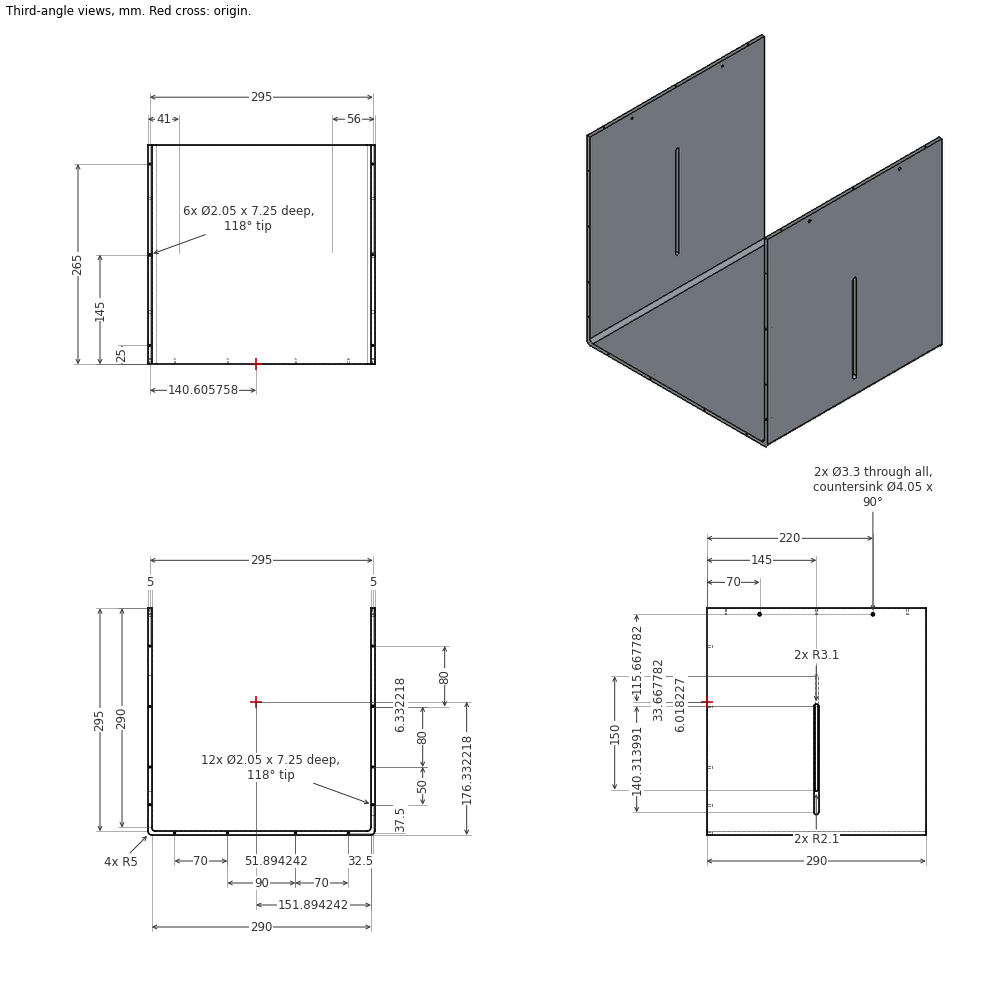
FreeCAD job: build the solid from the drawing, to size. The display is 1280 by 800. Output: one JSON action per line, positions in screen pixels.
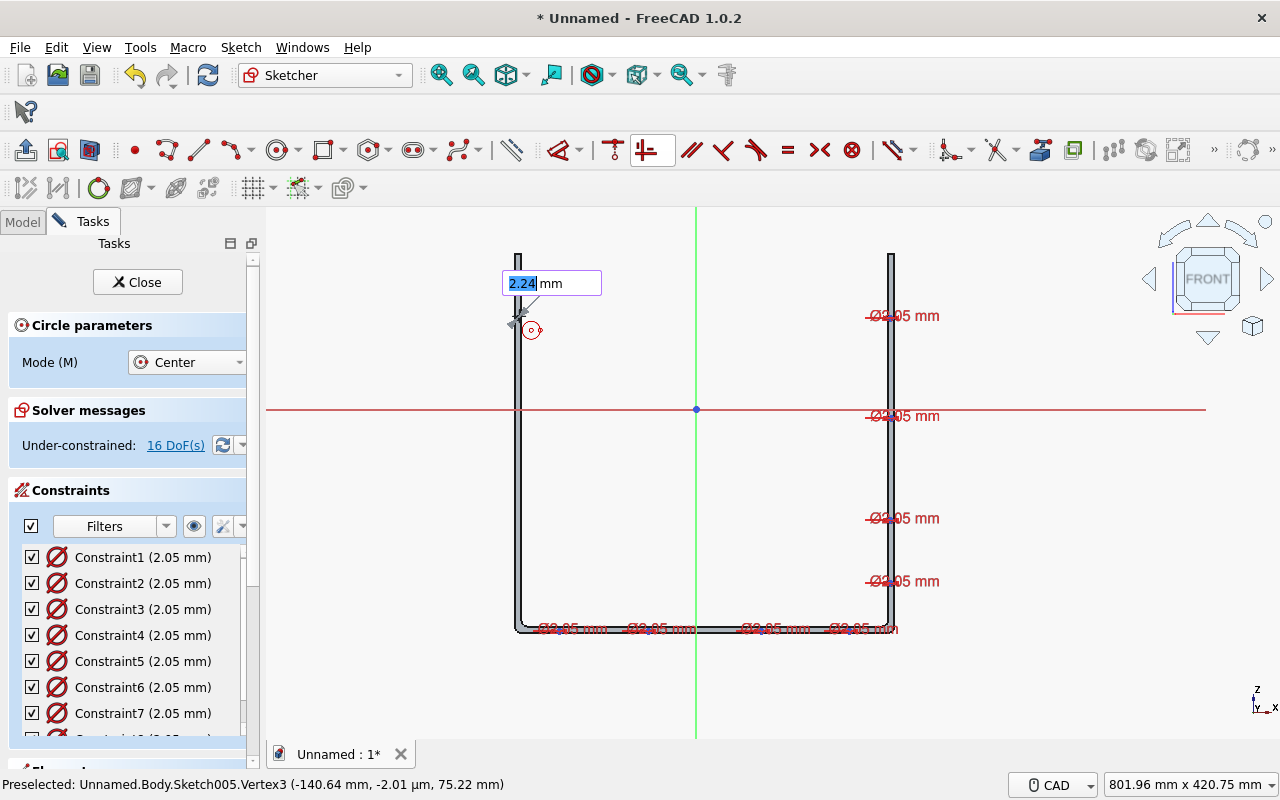
{"action": "type", "text": "2.05"}
{"action": "key", "text": "Return"}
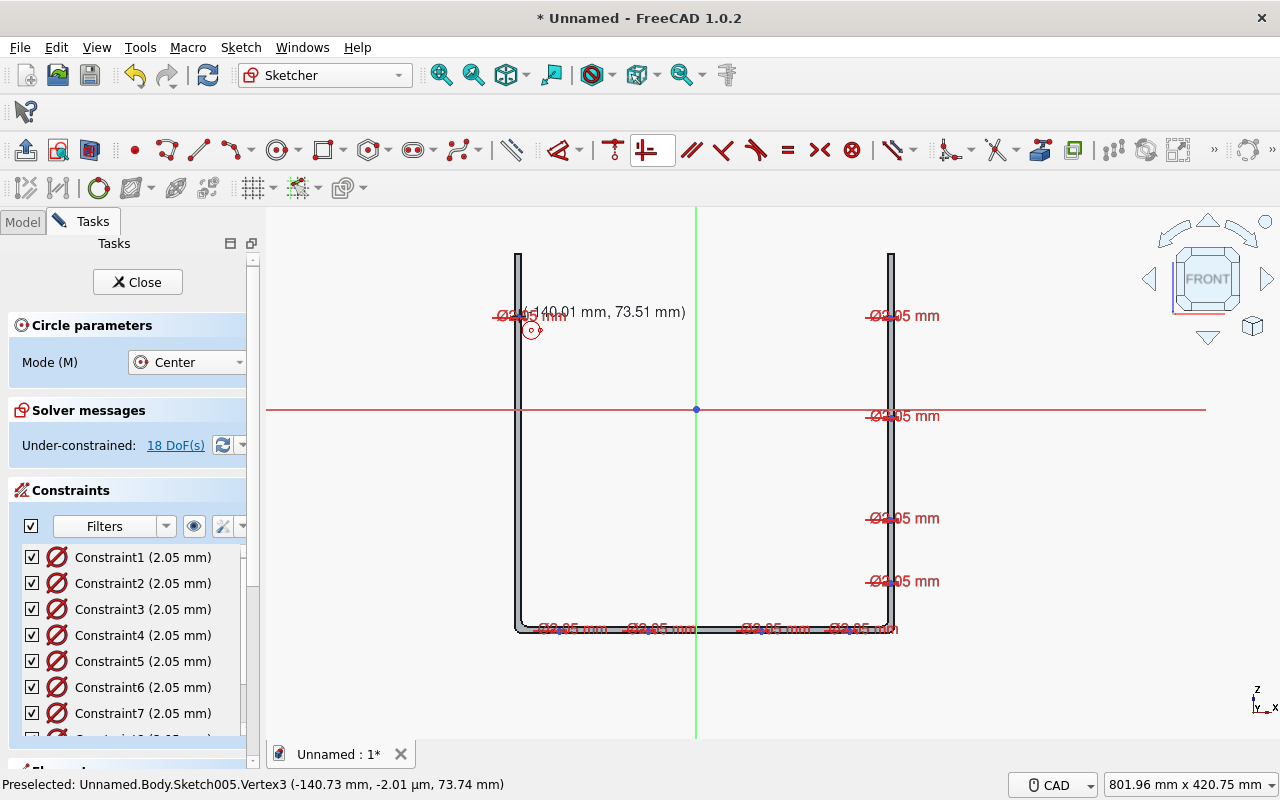
{"action": "scroll", "coordinate": [518, 418], "scroll_direction": "up", "scroll_amount": 15}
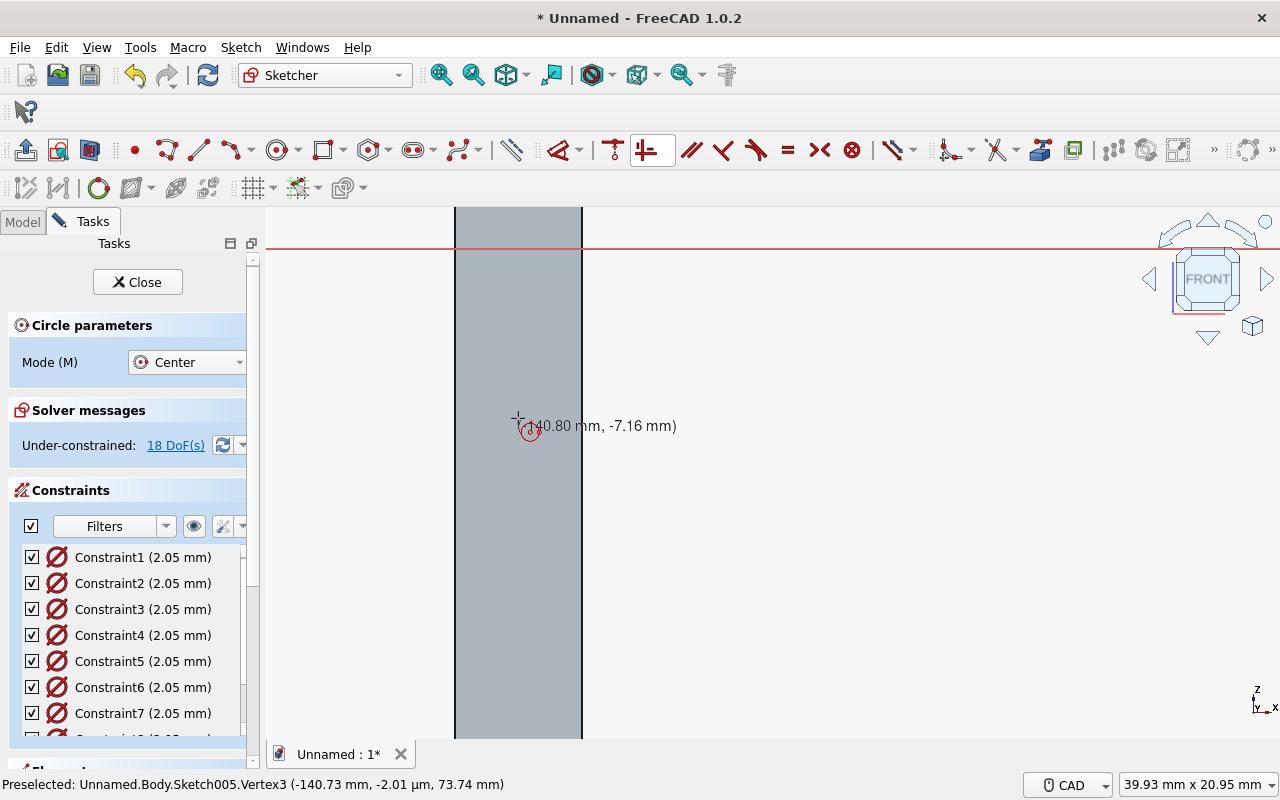
{"action": "scroll", "coordinate": [518, 418], "scroll_direction": "down", "scroll_amount": 15}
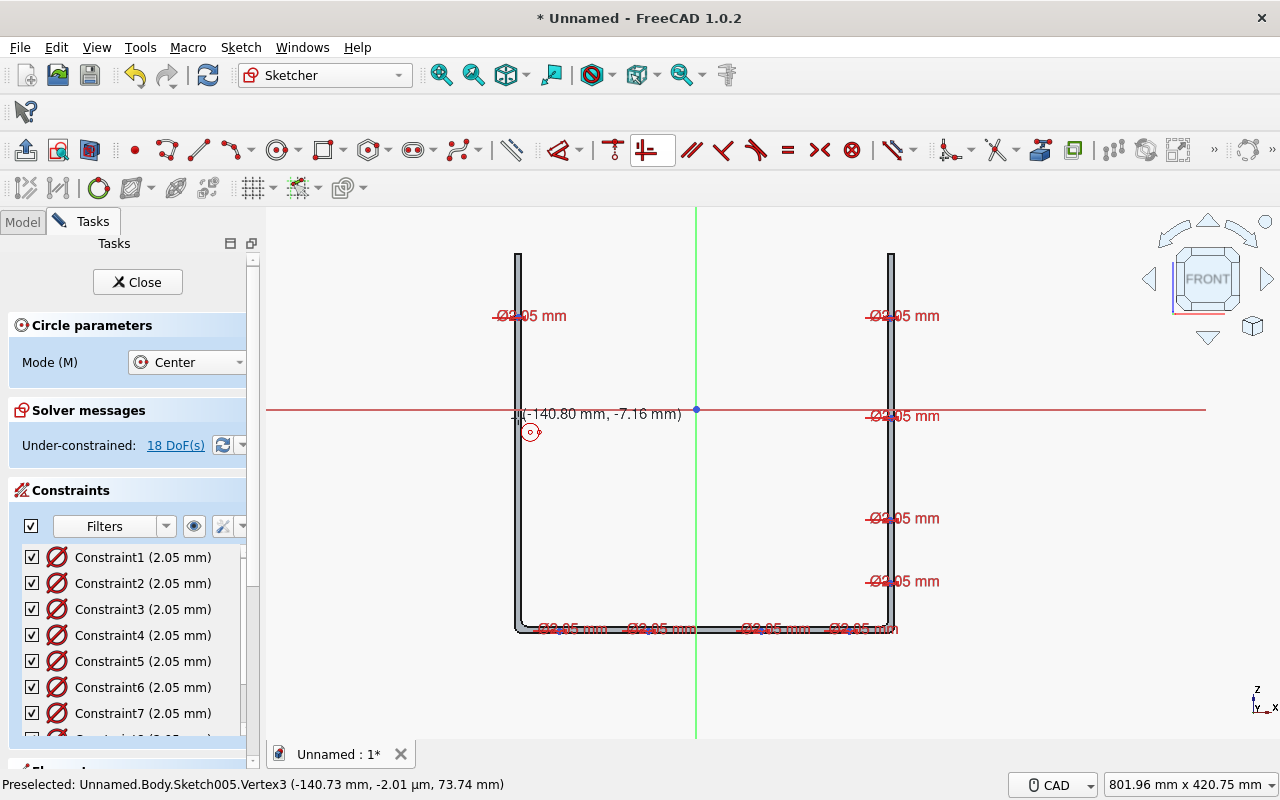
{"action": "scroll", "coordinate": [518, 418], "scroll_direction": "up", "scroll_amount": 4}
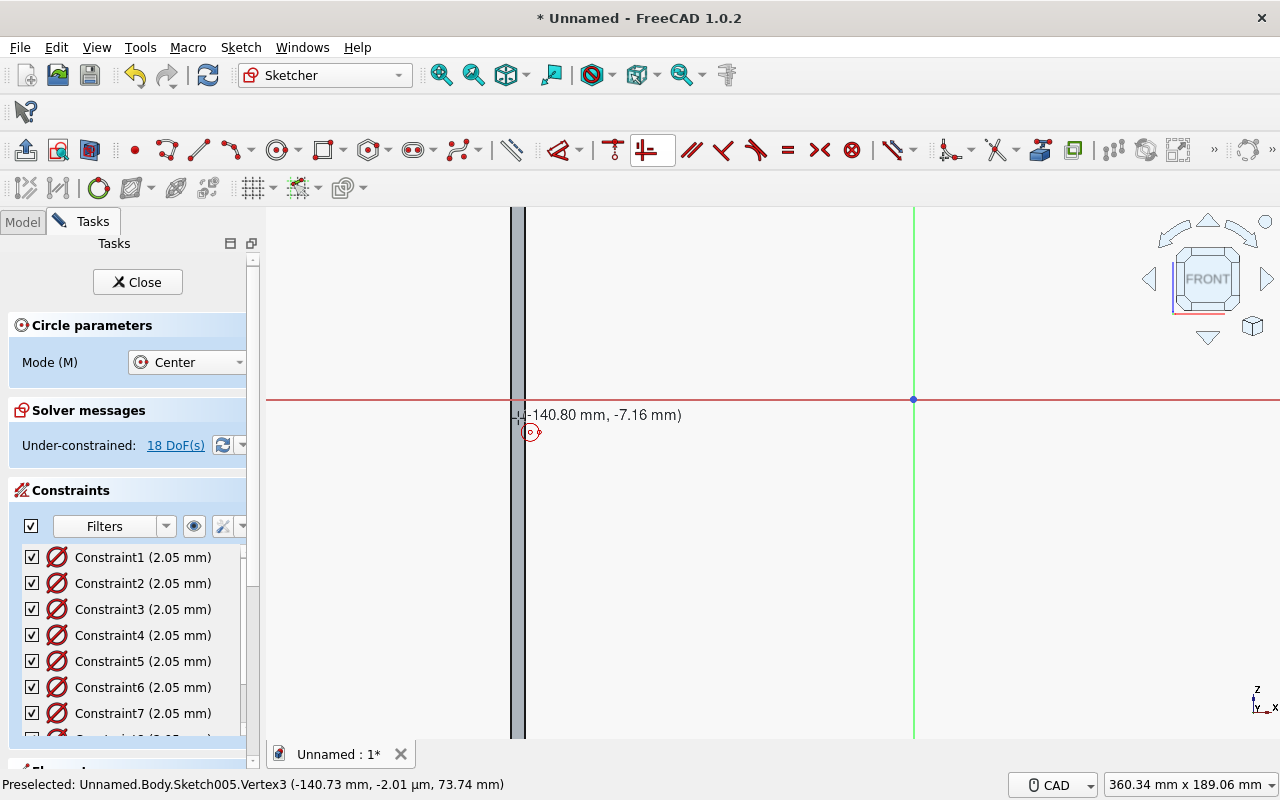
{"action": "left_click", "coordinate": [518, 417]}
{"action": "mouse_move", "coordinate": [520, 415]}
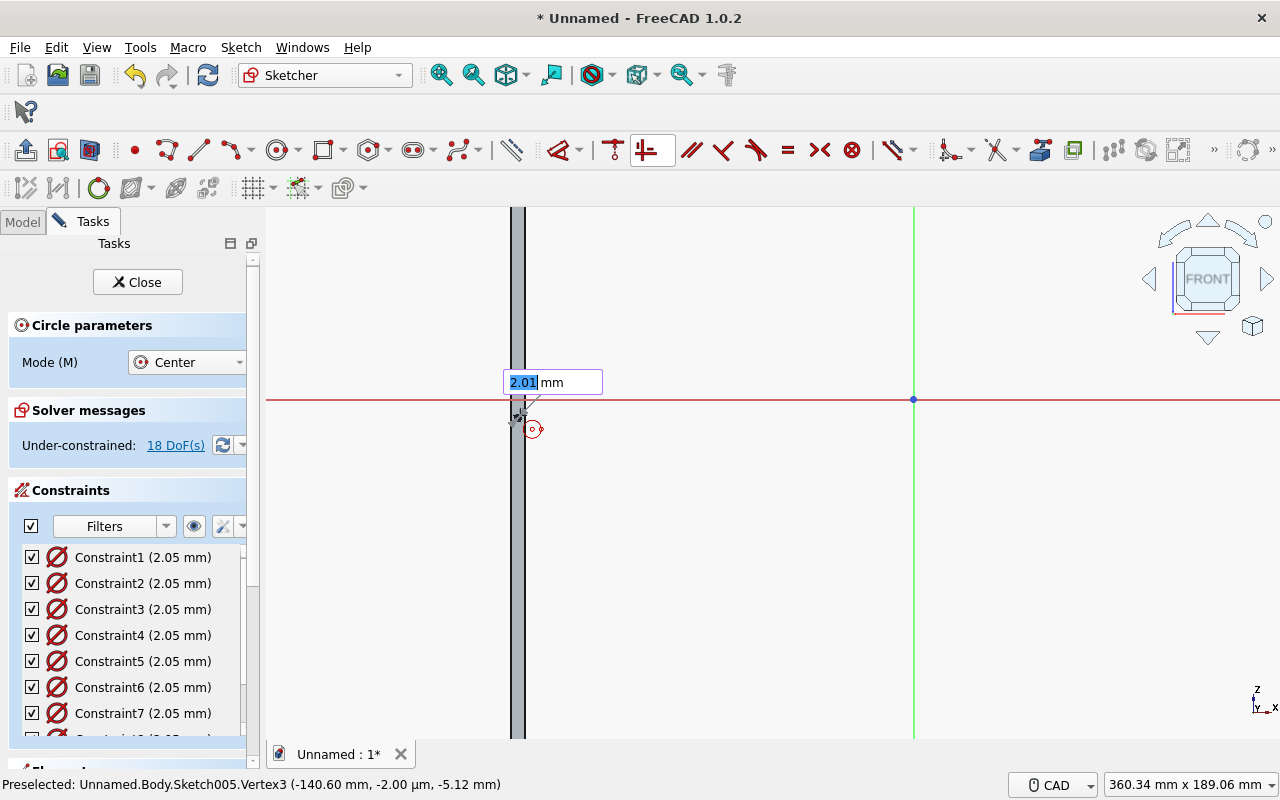
{"action": "type", "text": "2.05"}
{"action": "key", "text": "Return"}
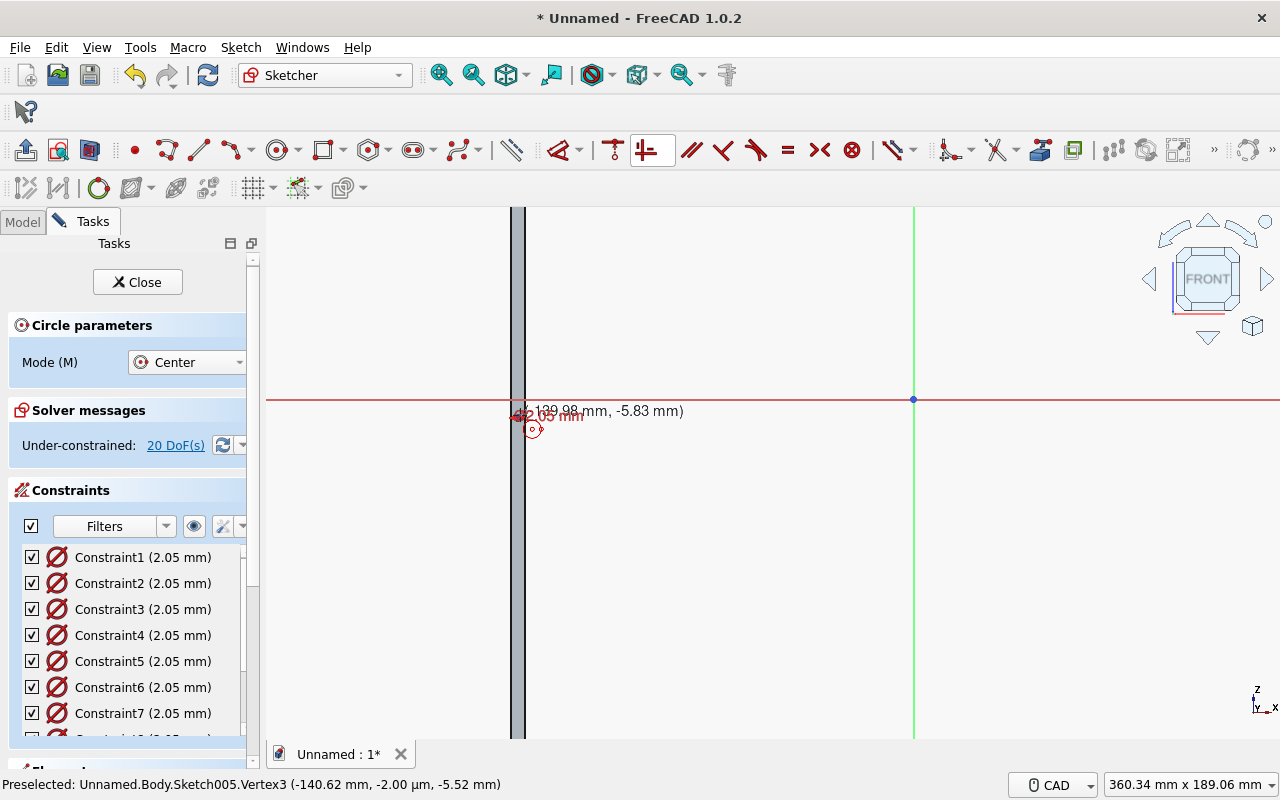
{"action": "scroll", "coordinate": [518, 643], "scroll_direction": "up", "scroll_amount": 11}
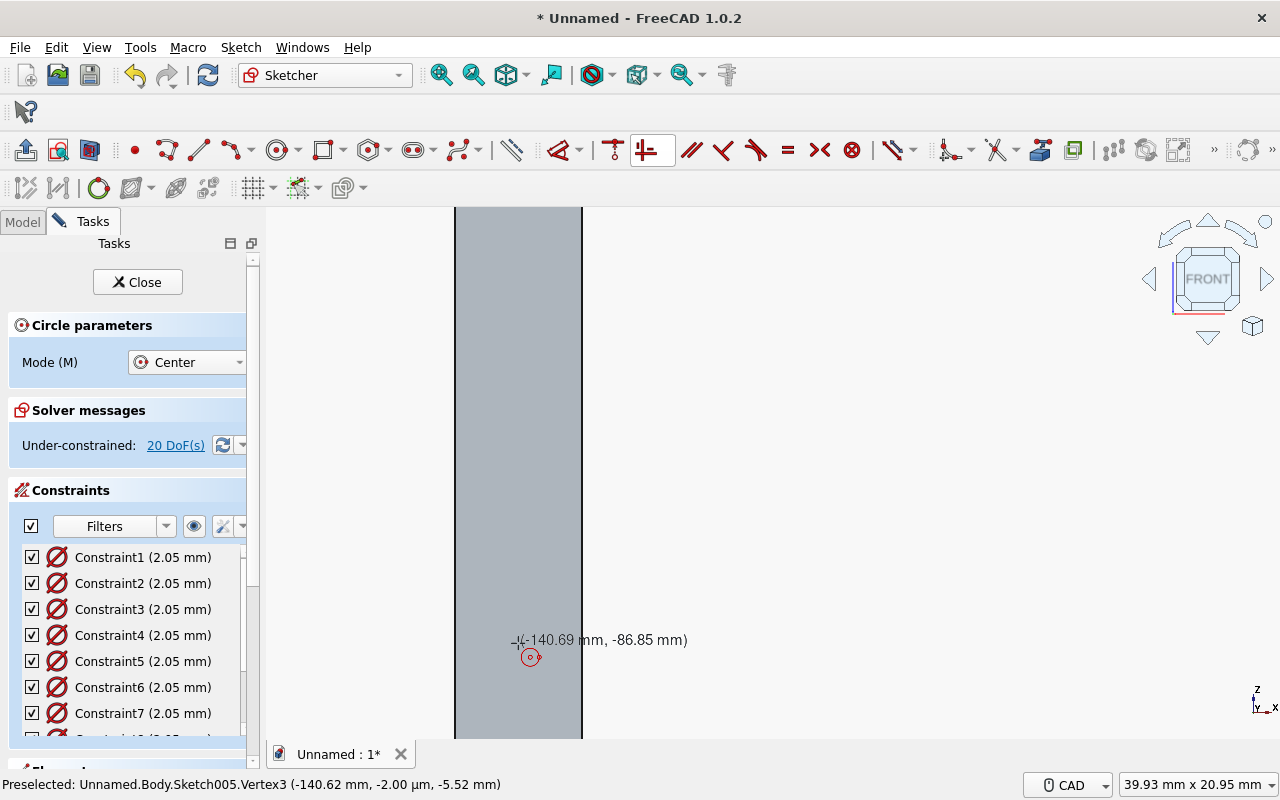
{"action": "scroll", "coordinate": [518, 513], "scroll_direction": "down", "scroll_amount": 15}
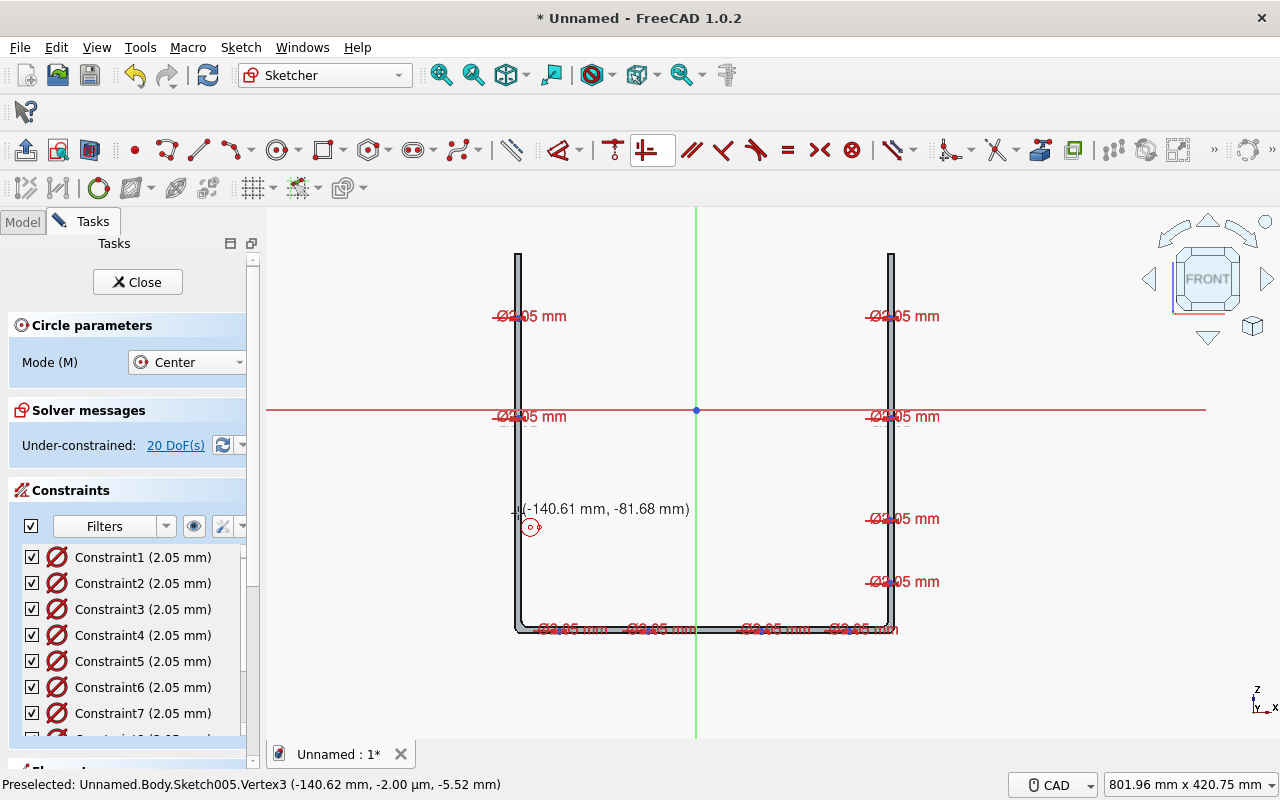
{"action": "left_click", "coordinate": [518, 519]}
{"action": "mouse_move", "coordinate": [519, 519]}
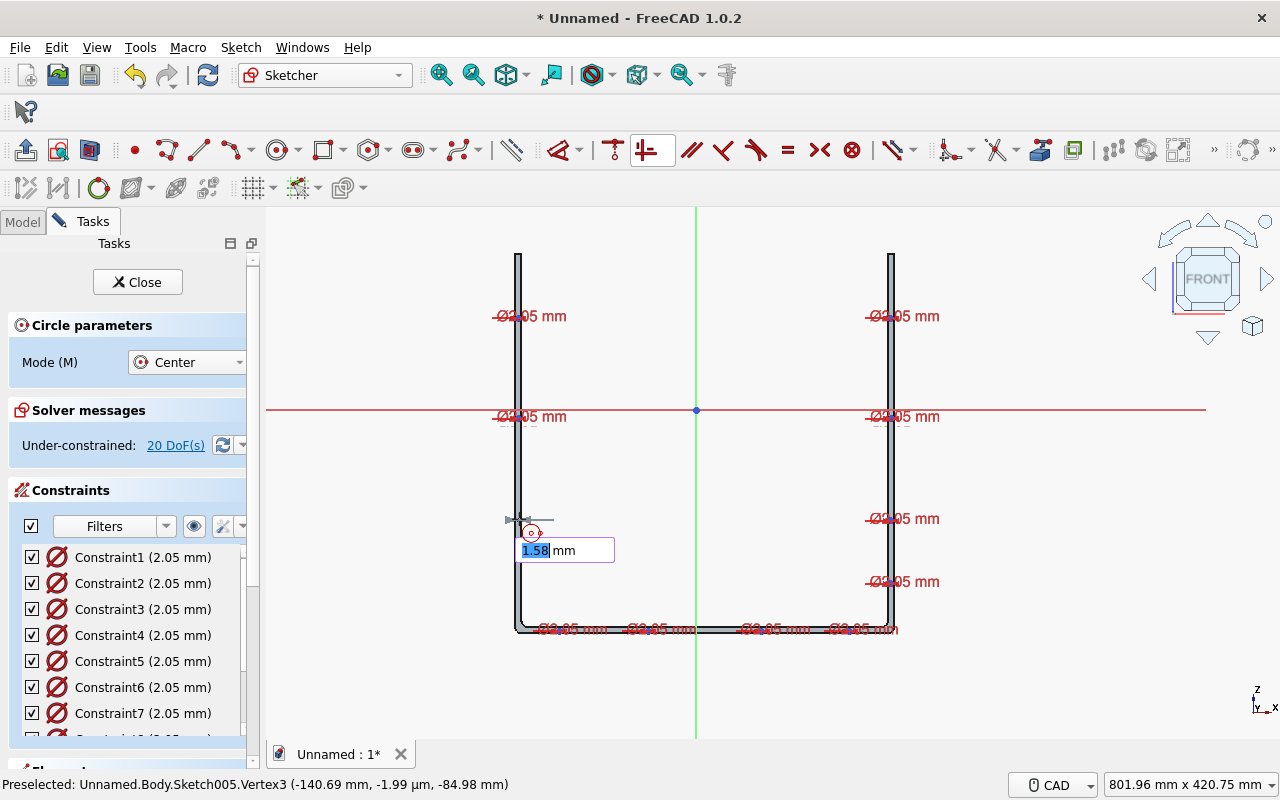
{"action": "type", "text": "2.05"}
{"action": "key", "text": "Return"}